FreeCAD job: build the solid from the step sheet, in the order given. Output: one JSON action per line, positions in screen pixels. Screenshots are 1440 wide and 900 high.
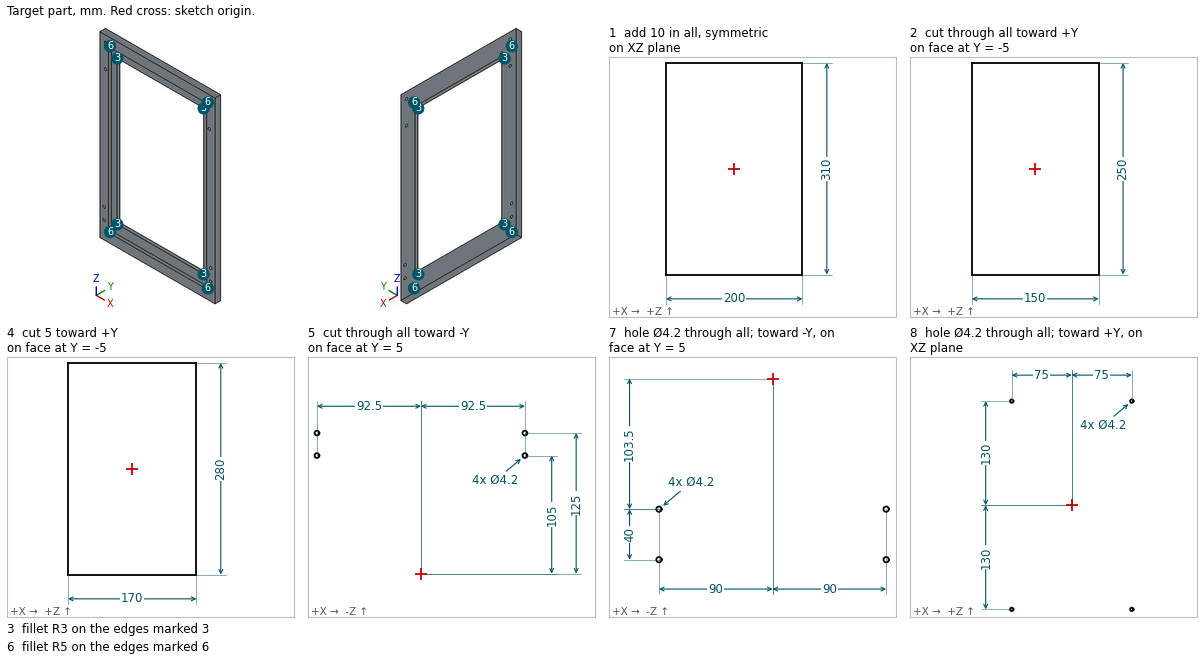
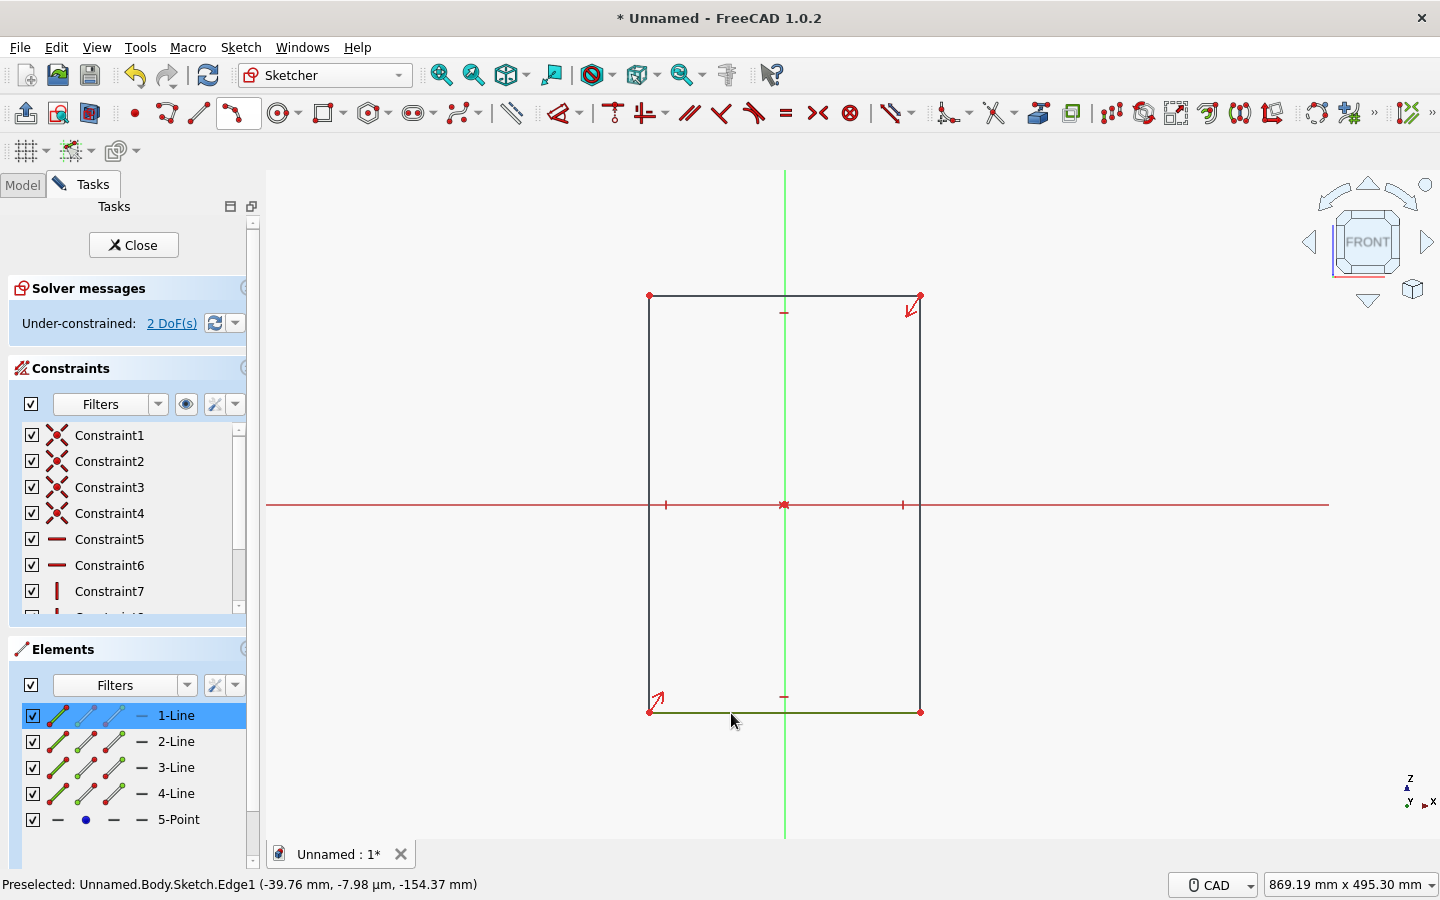
{"action": "left_click", "coordinate": [582, 114]}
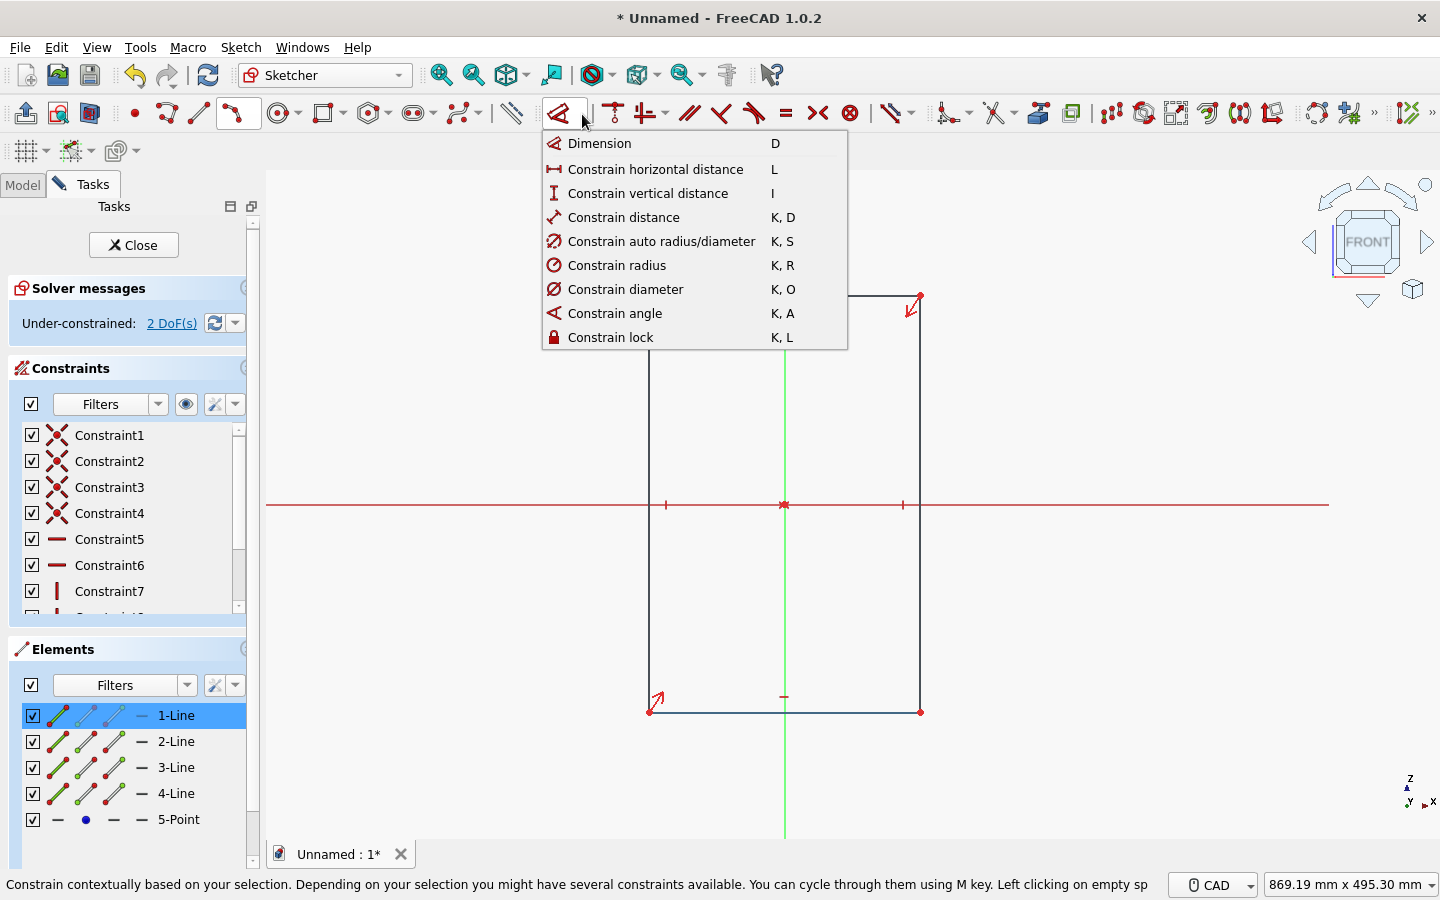
{"action": "left_click", "coordinate": [695, 169]}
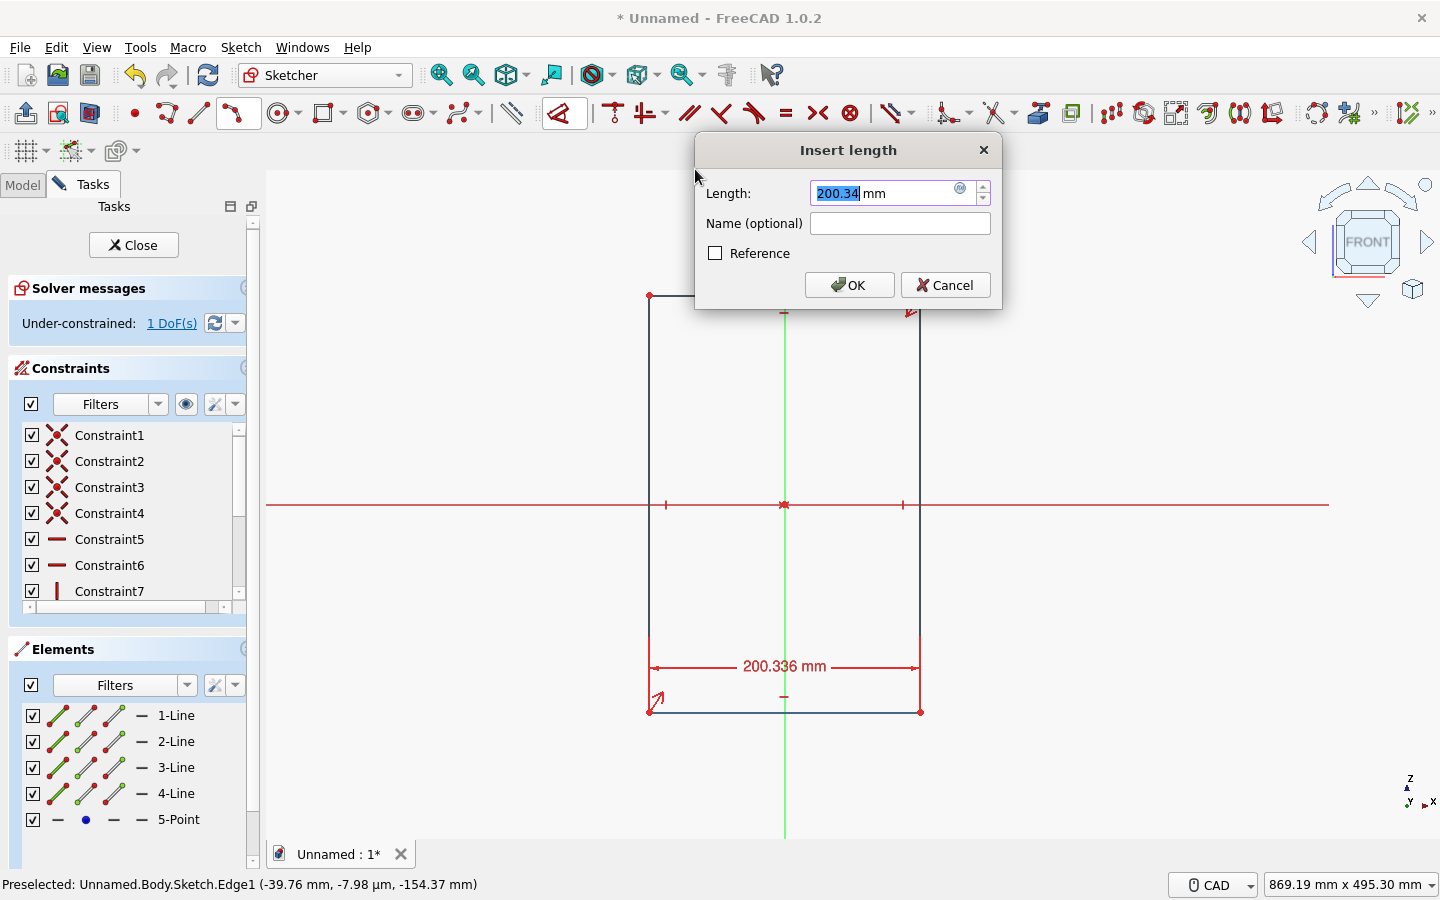
{"action": "type", "text": "200"}
{"action": "key", "text": "Return"}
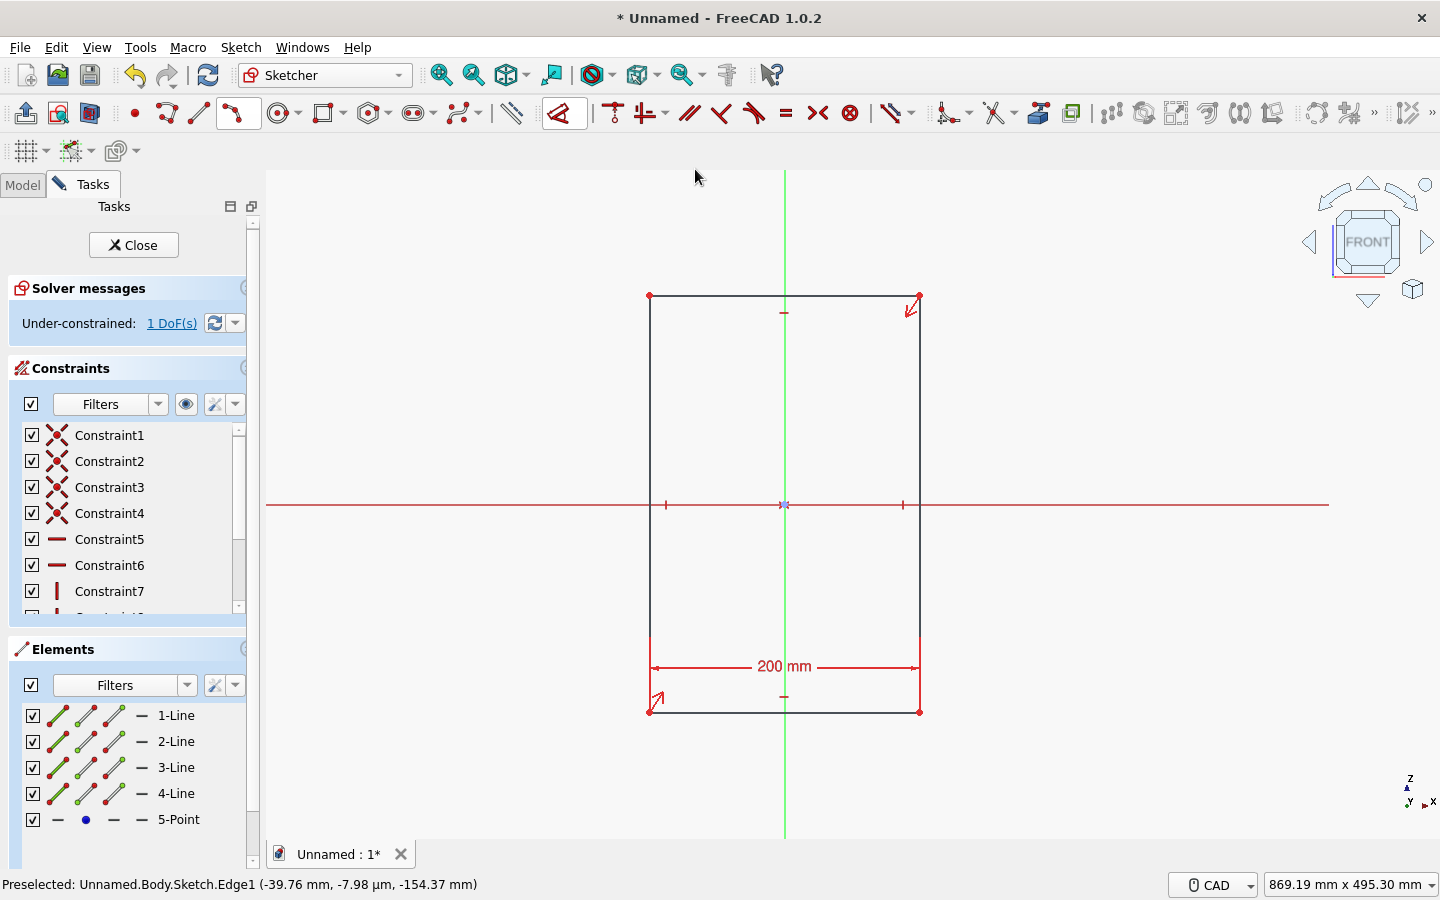
{"action": "left_click", "coordinate": [920, 588]}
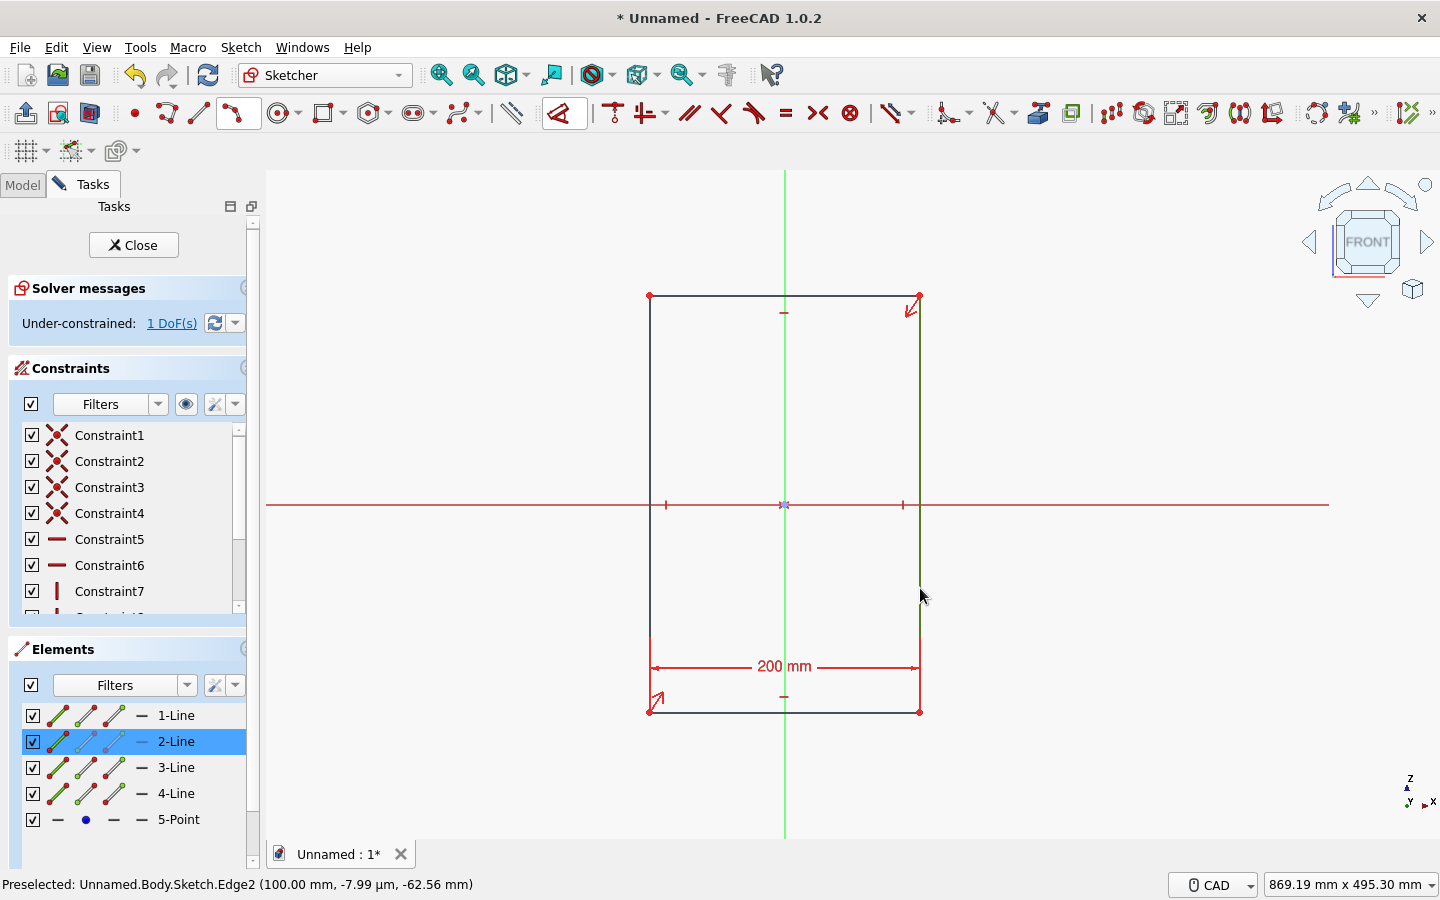
{"action": "key", "text": "i"}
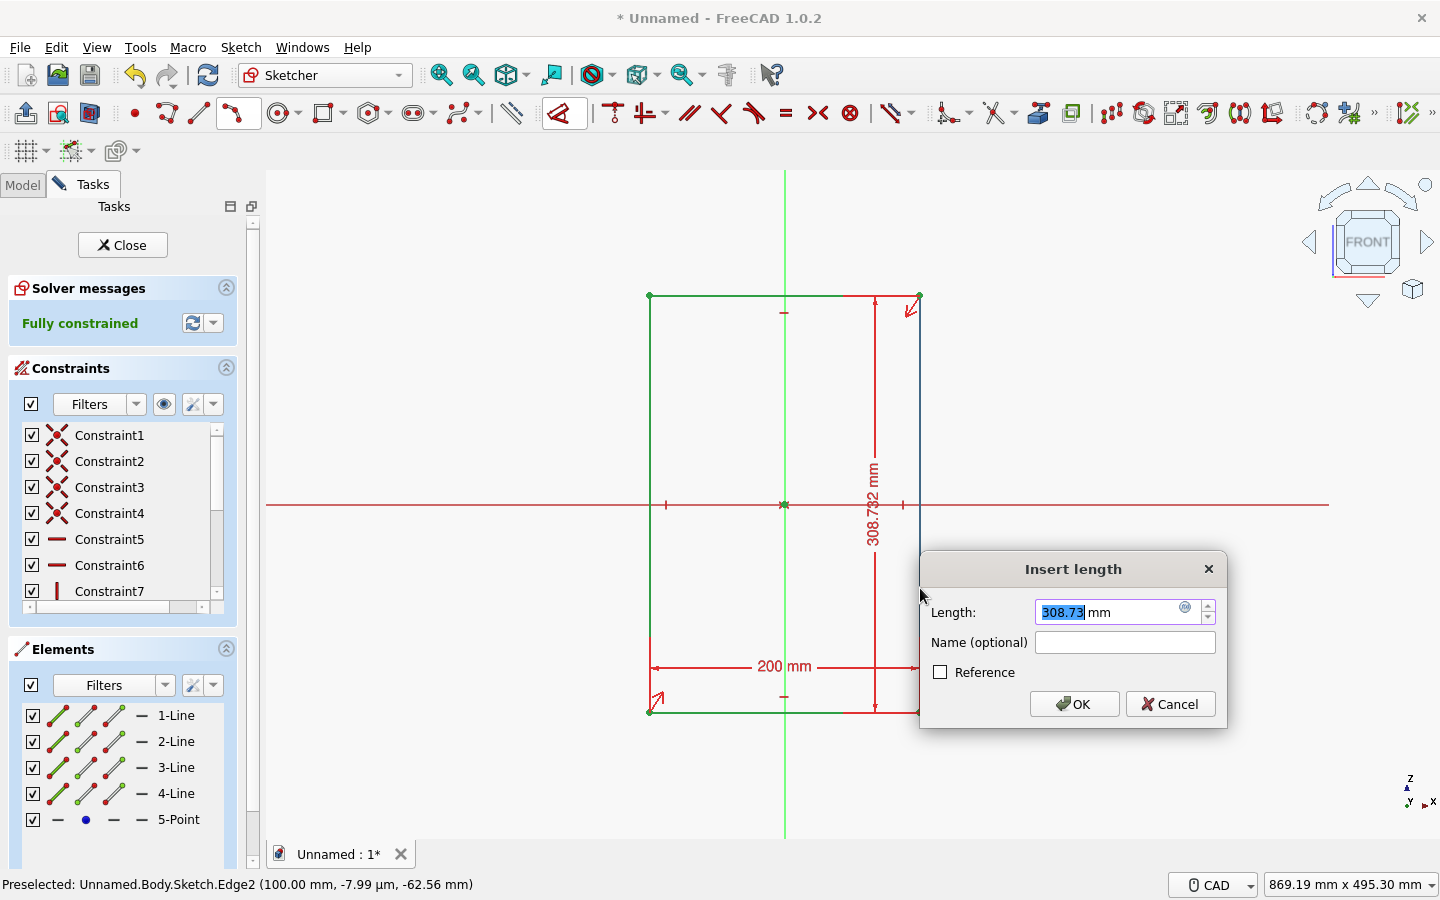
{"action": "type", "text": "310"}
{"action": "key", "text": "Return"}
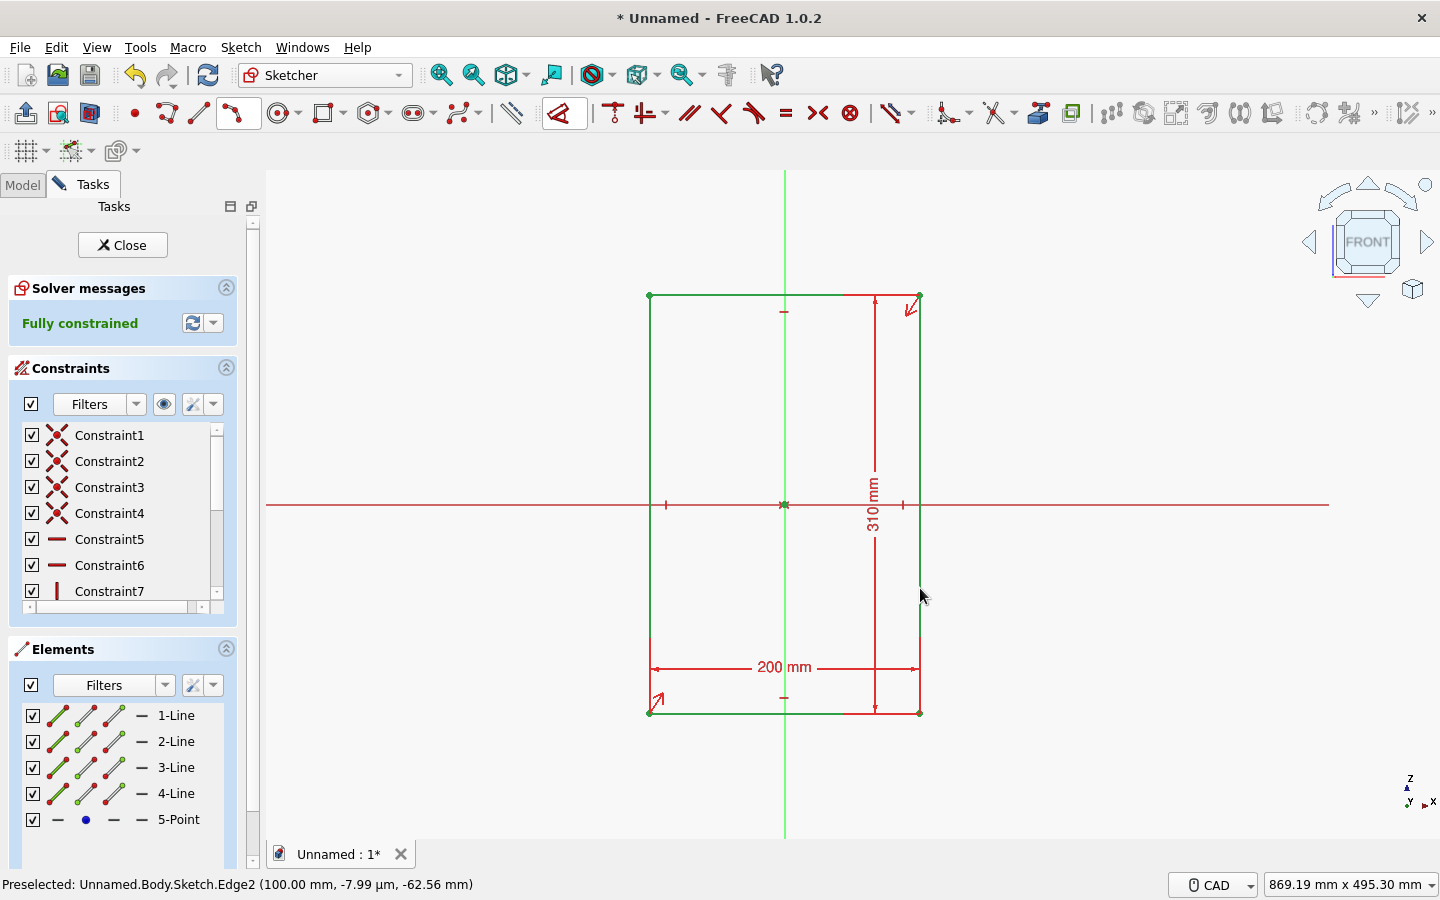
{"action": "left_click", "coordinate": [123, 245]}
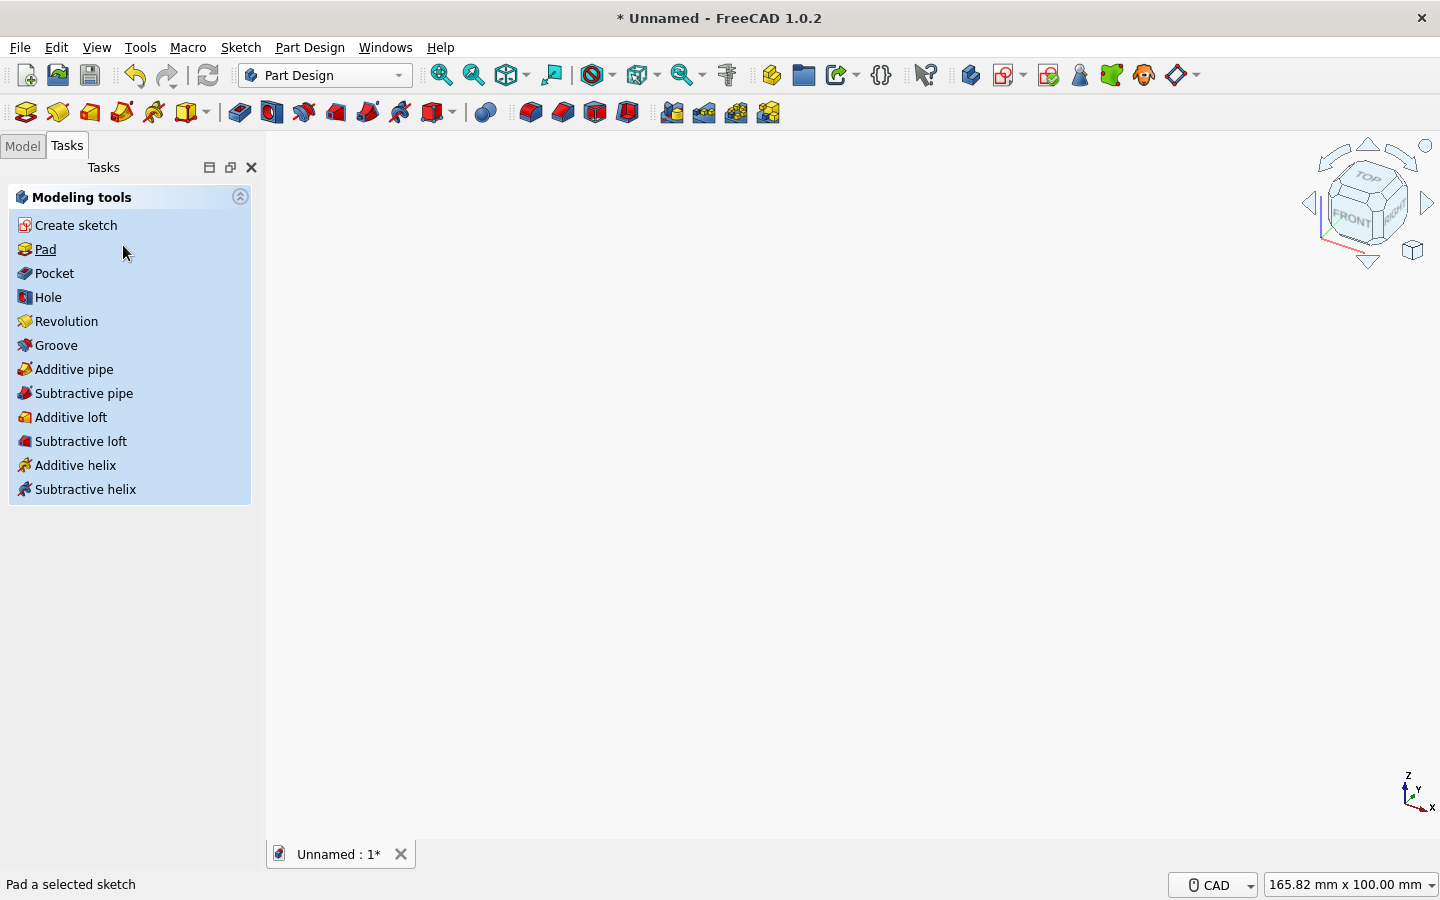
{"action": "left_click", "coordinate": [26, 112]}